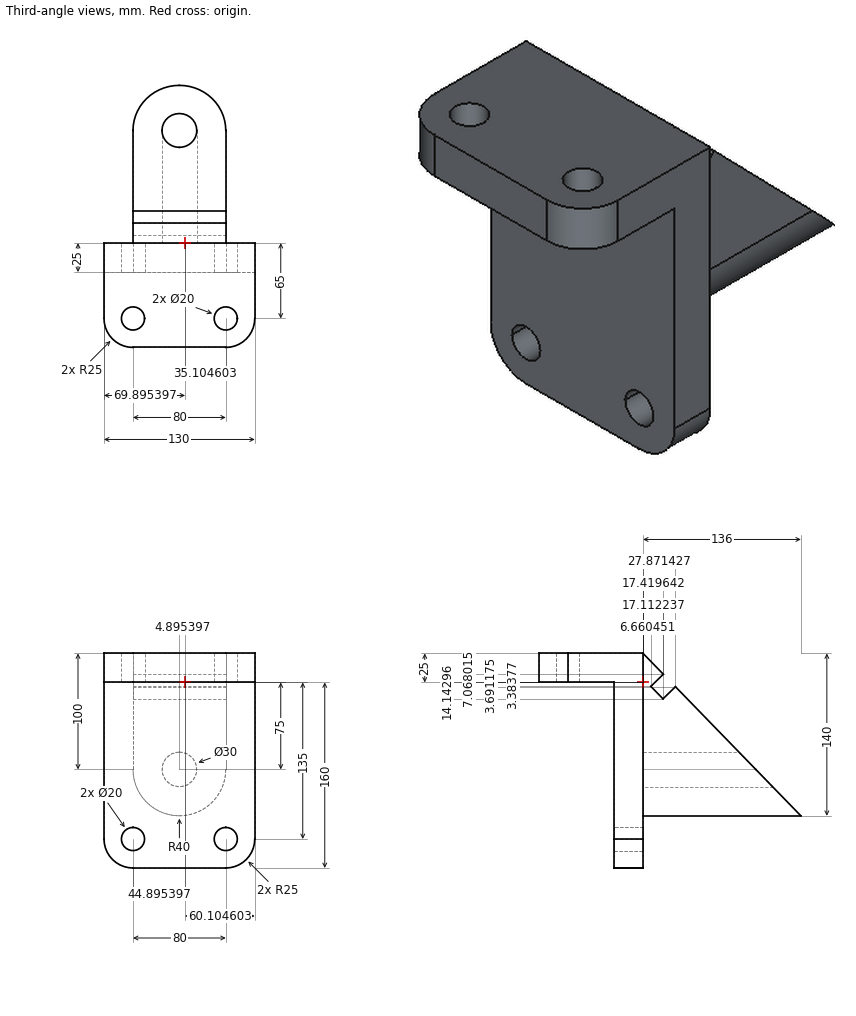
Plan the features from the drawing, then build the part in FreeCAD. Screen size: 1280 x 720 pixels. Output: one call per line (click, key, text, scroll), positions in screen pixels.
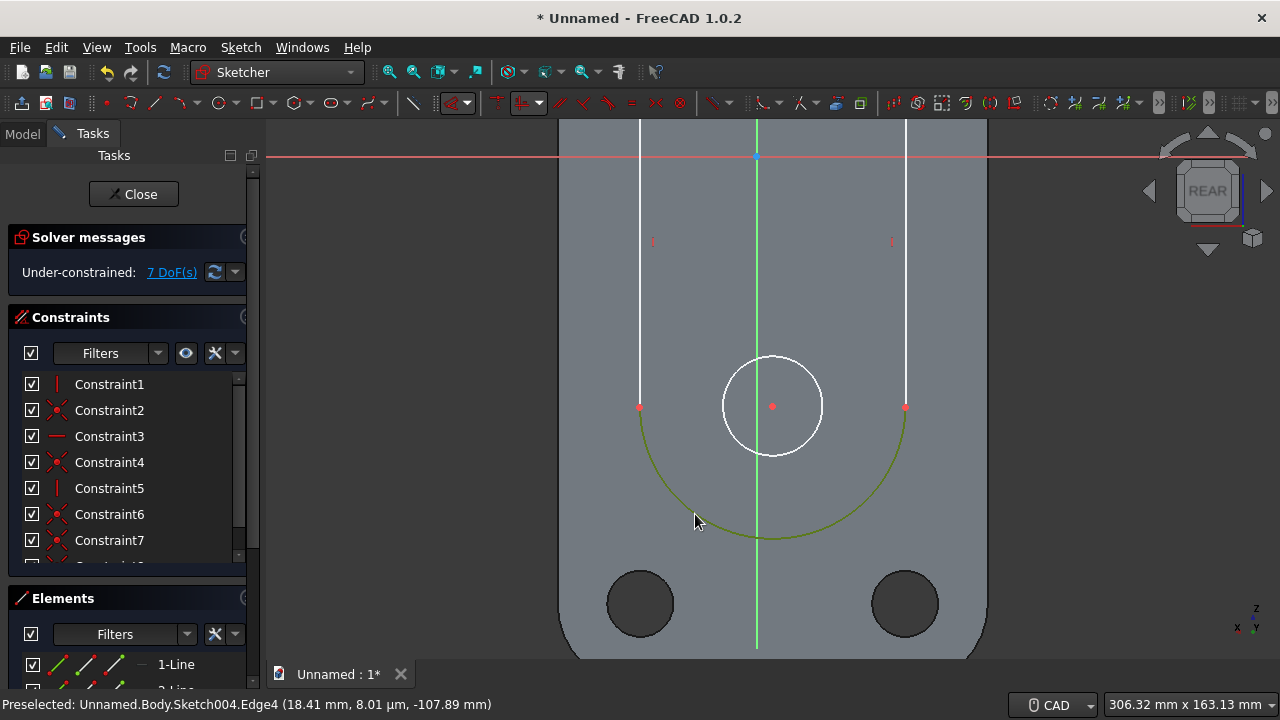
key(k)
key(r)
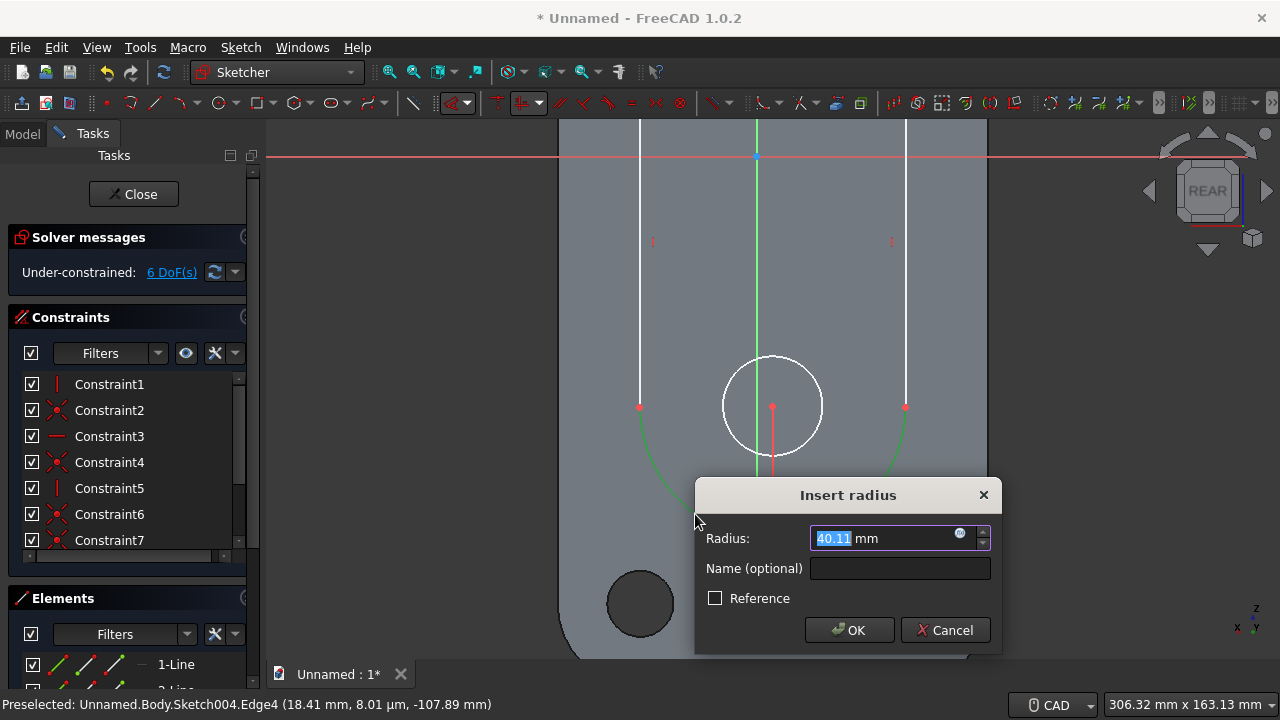
text(40)
key(Return)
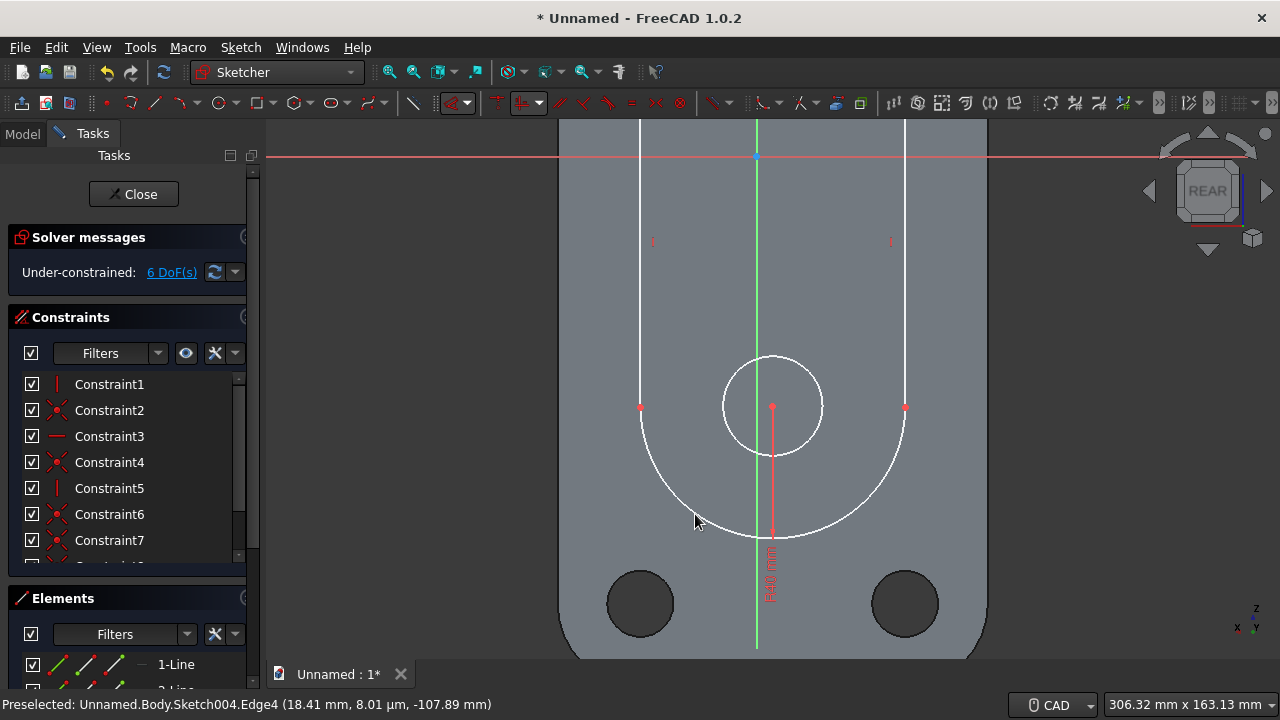
click(808, 371)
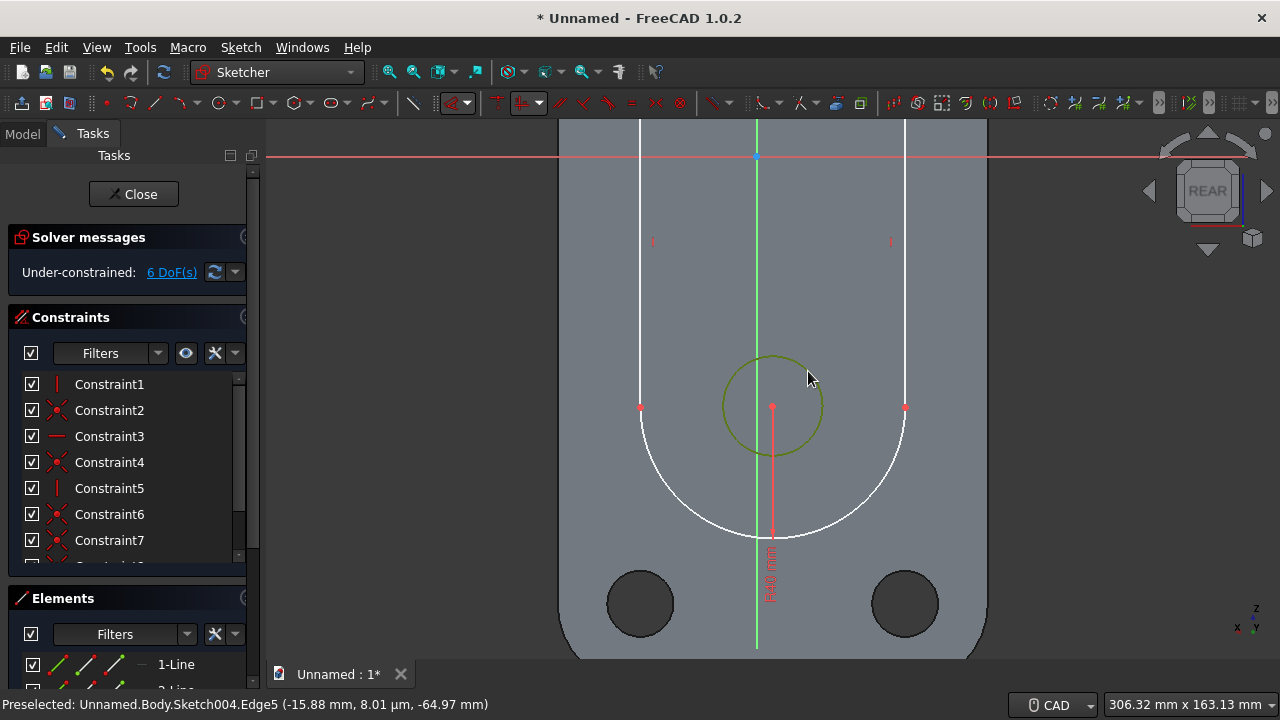
click(470, 104)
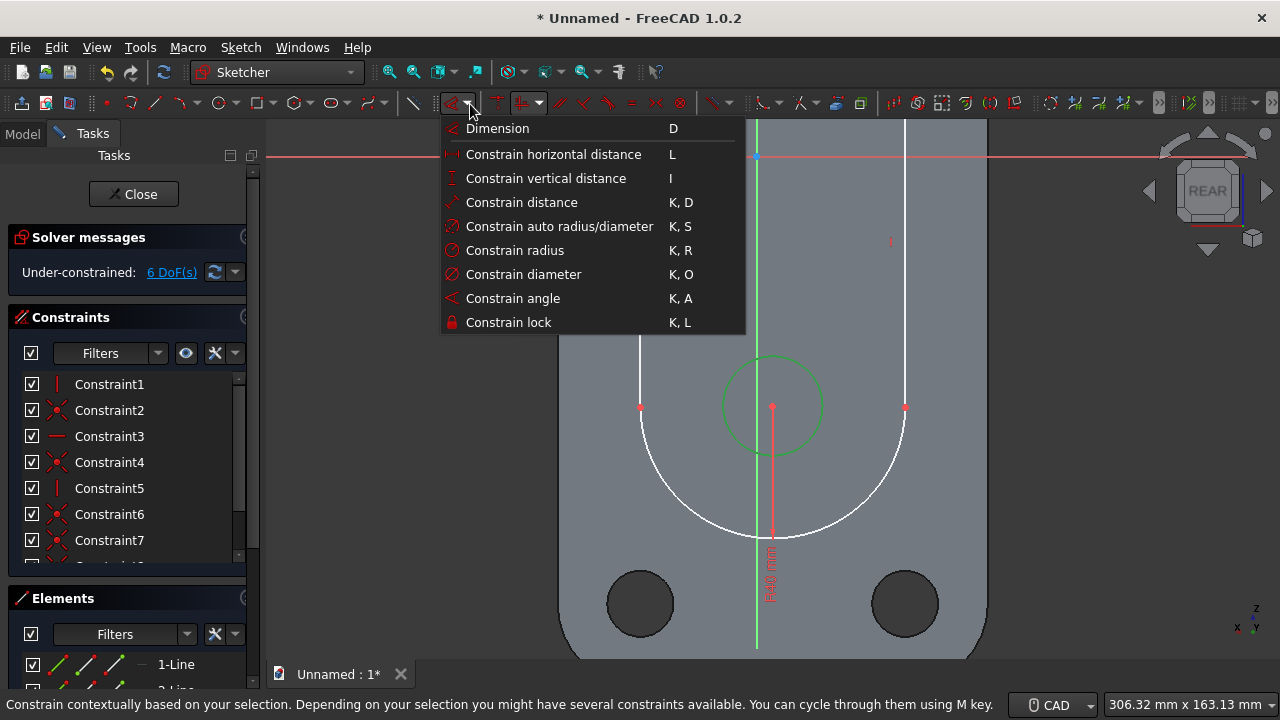
click(593, 274)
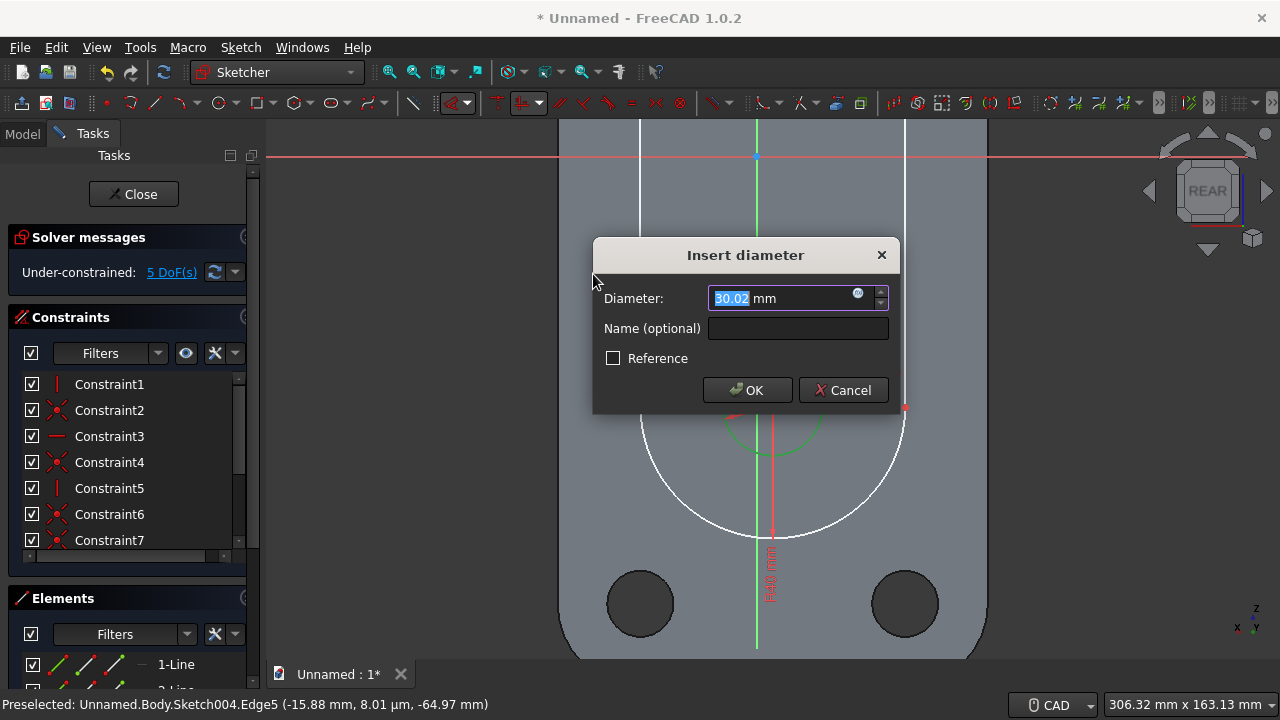
text(30)
key(Return)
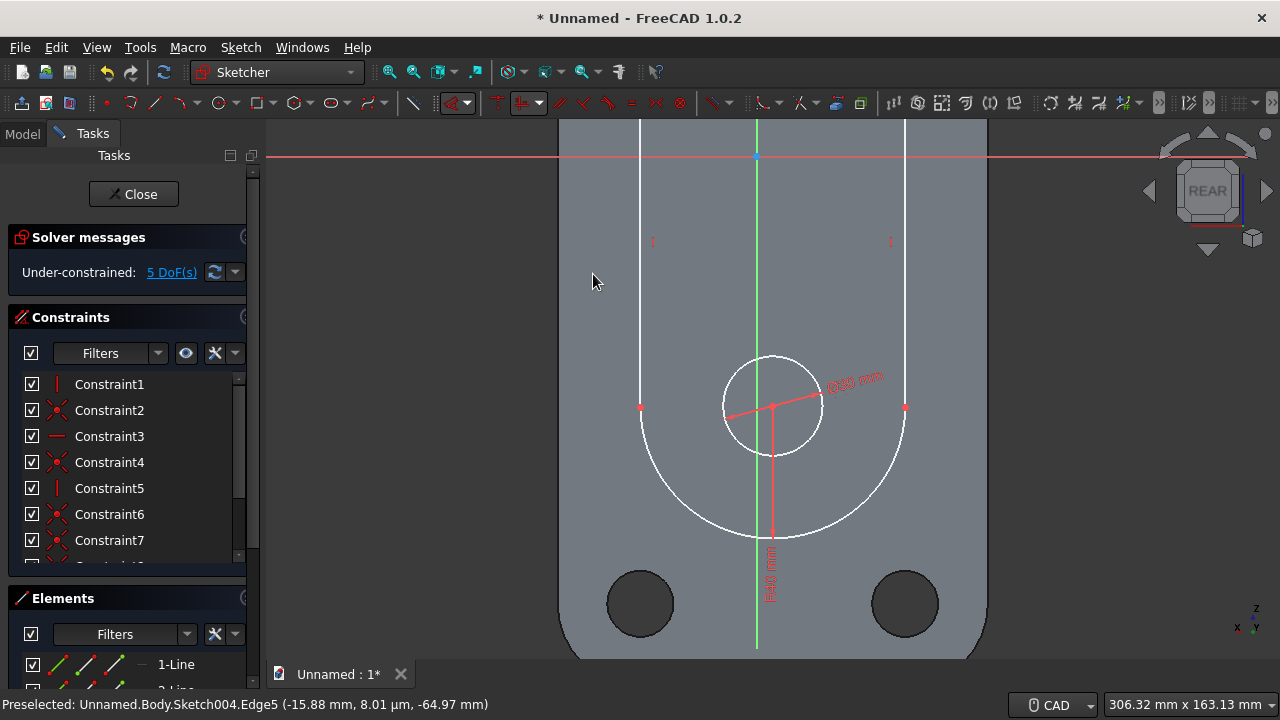
click(773, 406)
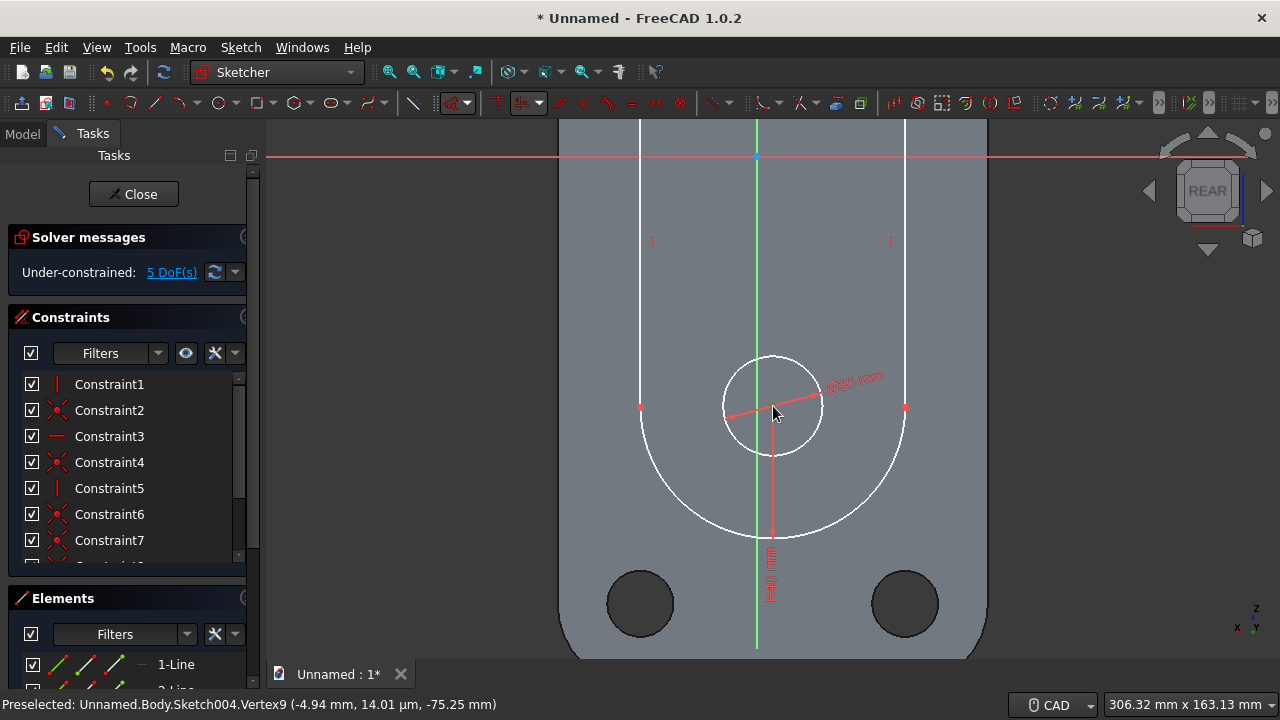
click(470, 104)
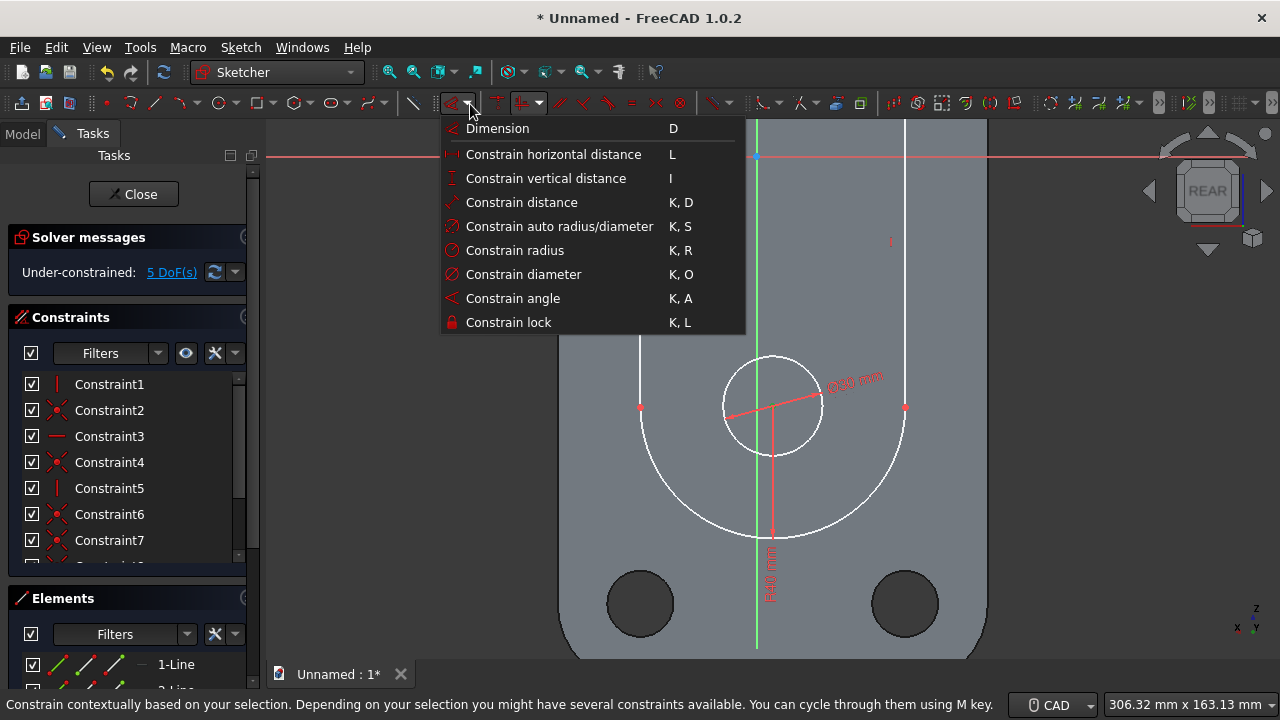
click(593, 178)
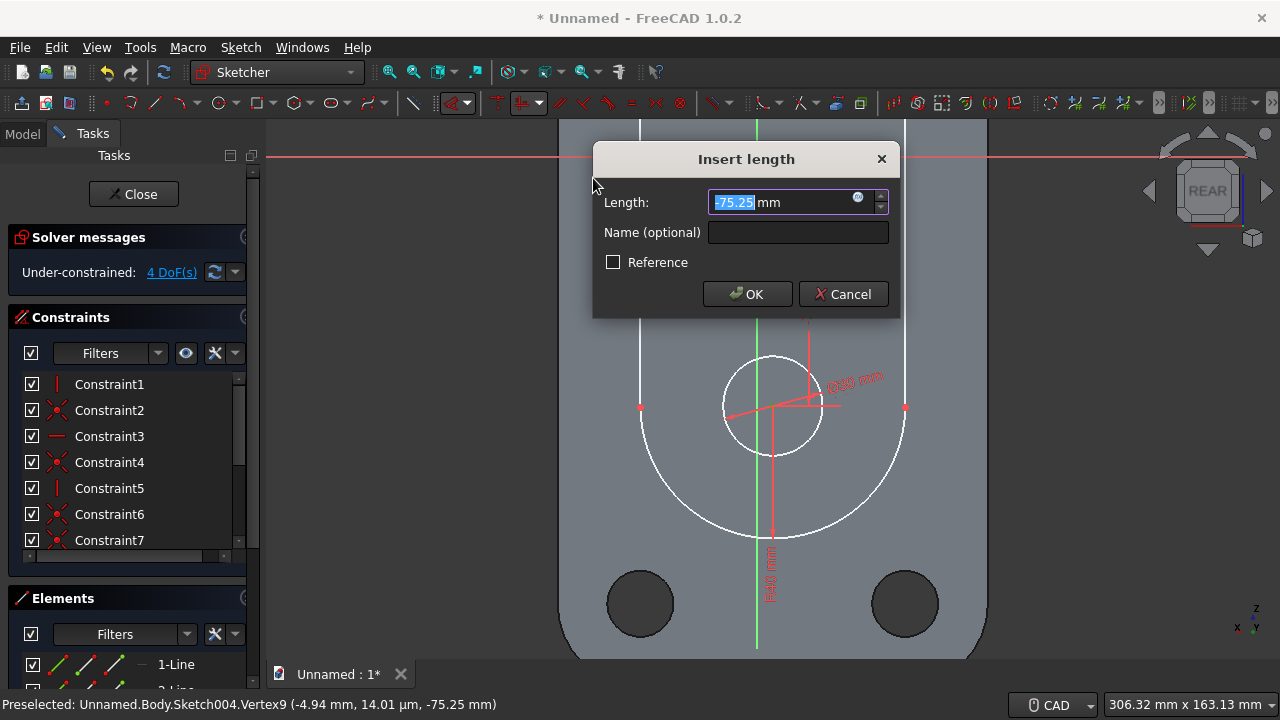
text(-75)
key(Return)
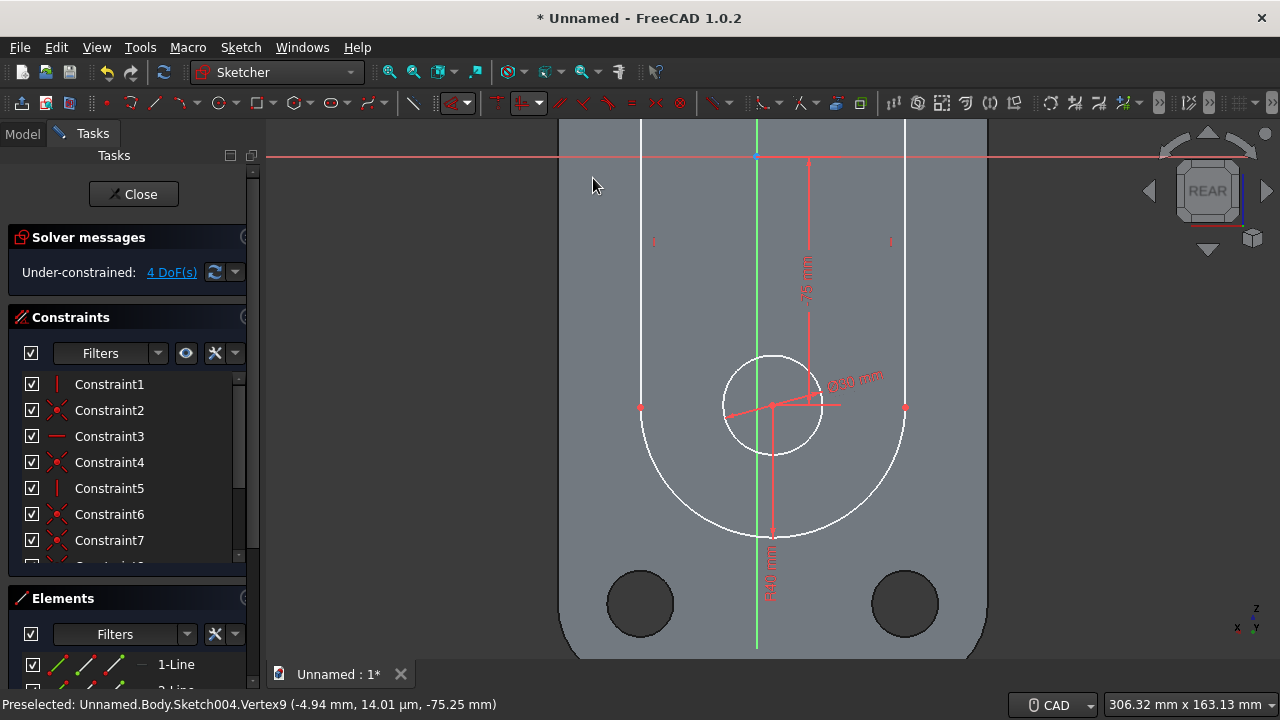
click(905, 308)